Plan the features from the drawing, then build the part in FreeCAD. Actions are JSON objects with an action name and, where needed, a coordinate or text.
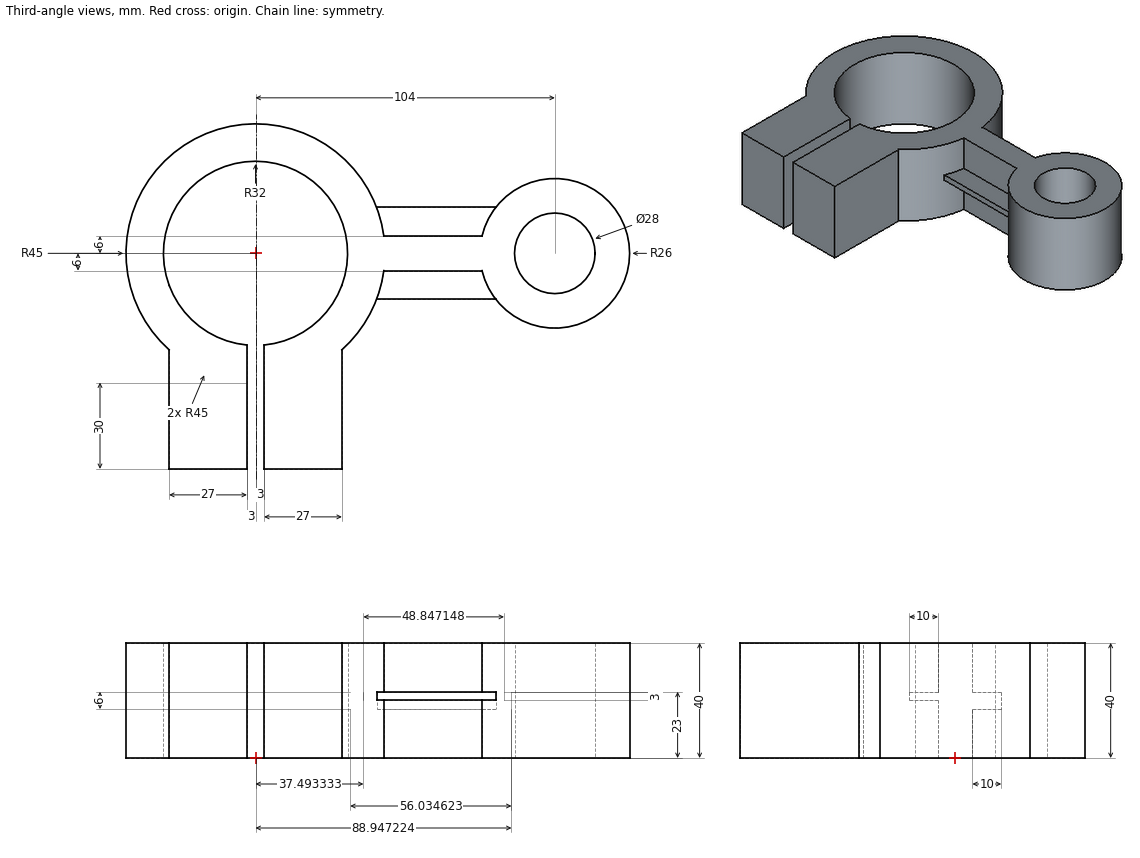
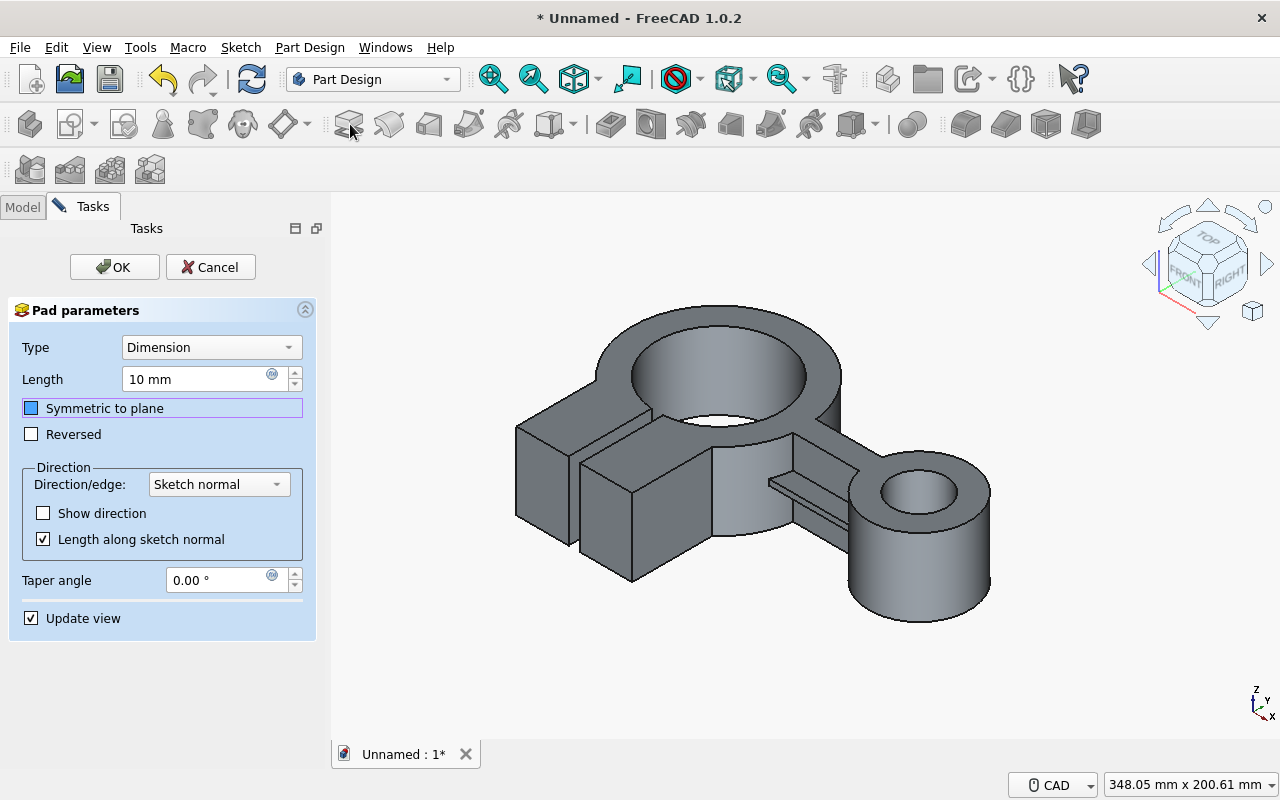
{"action": "left_click", "coordinate": [115, 267]}